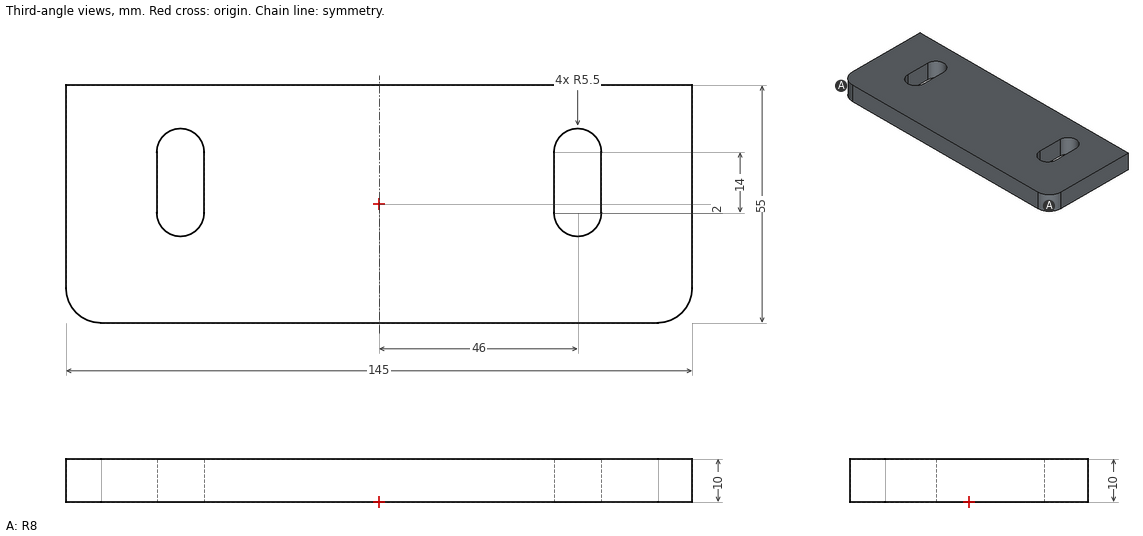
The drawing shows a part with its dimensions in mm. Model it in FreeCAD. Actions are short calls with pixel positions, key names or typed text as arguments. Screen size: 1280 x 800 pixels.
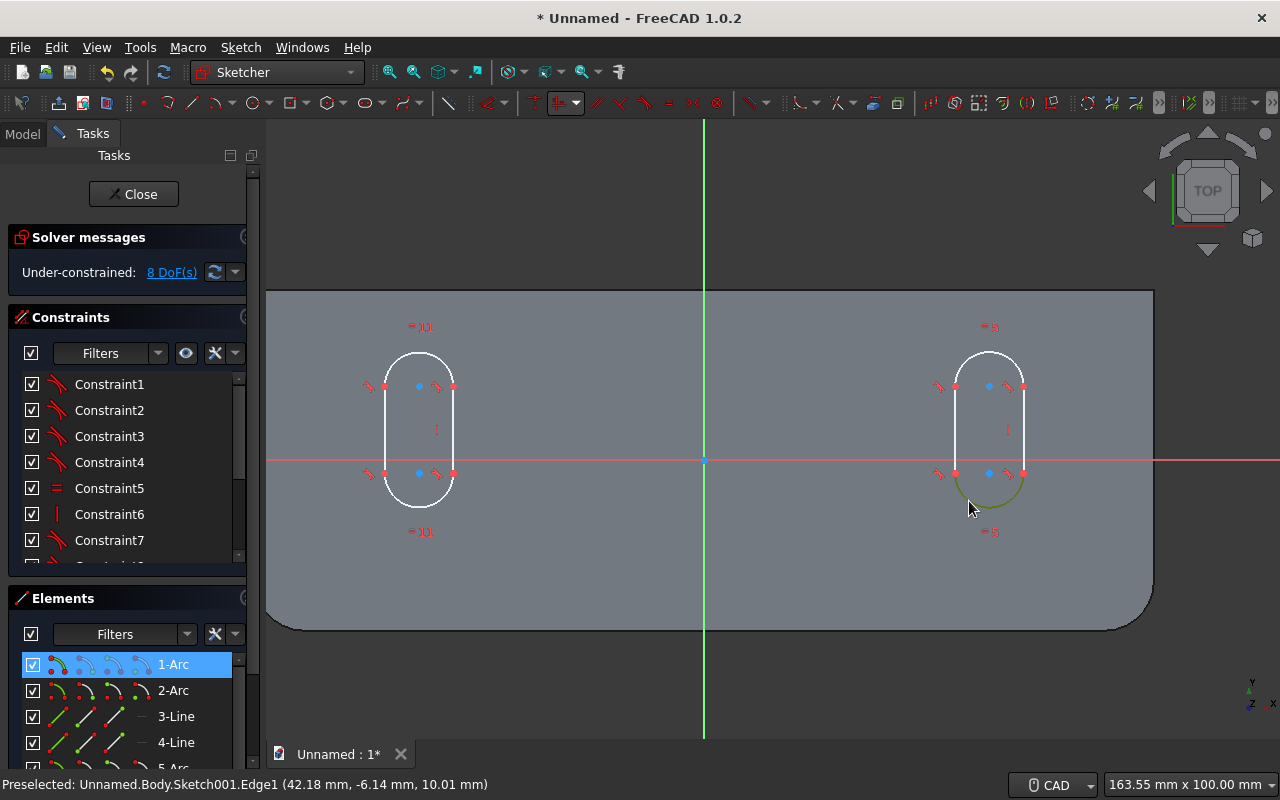
click(399, 501)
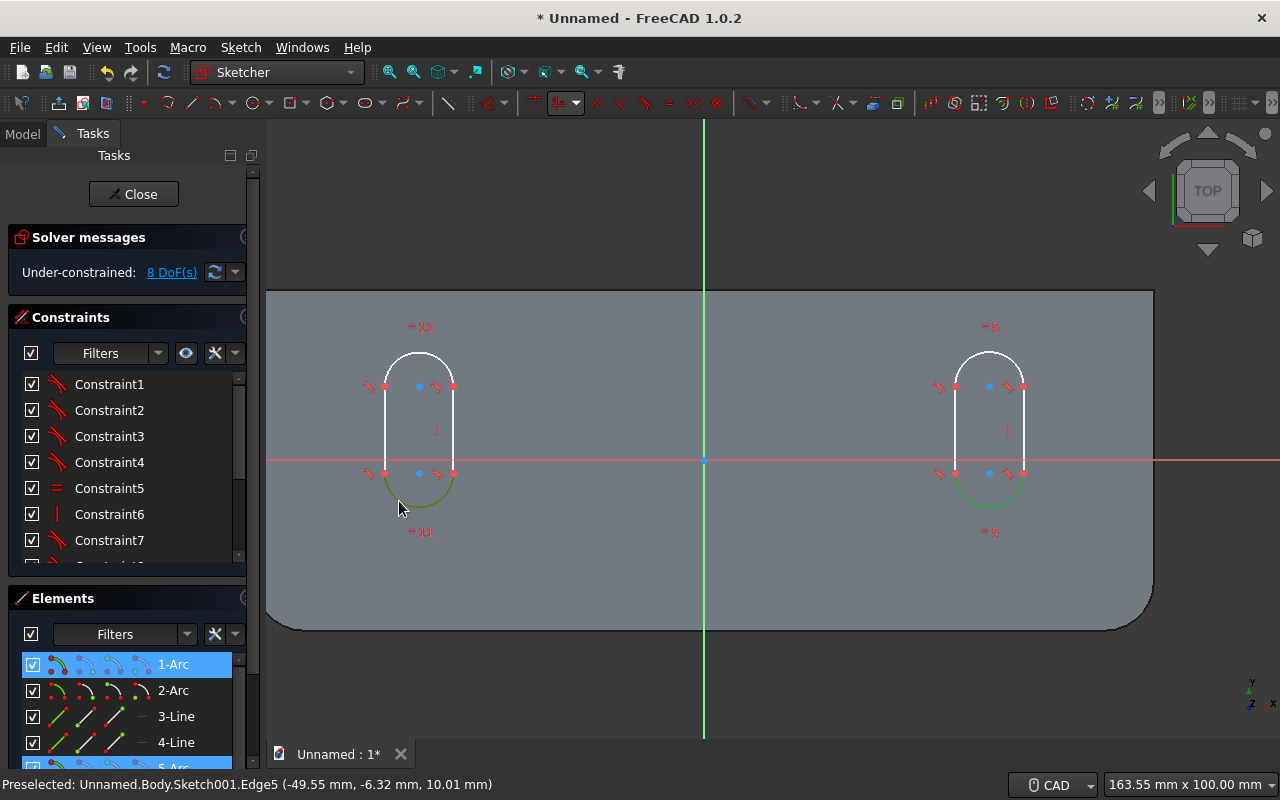
click(670, 104)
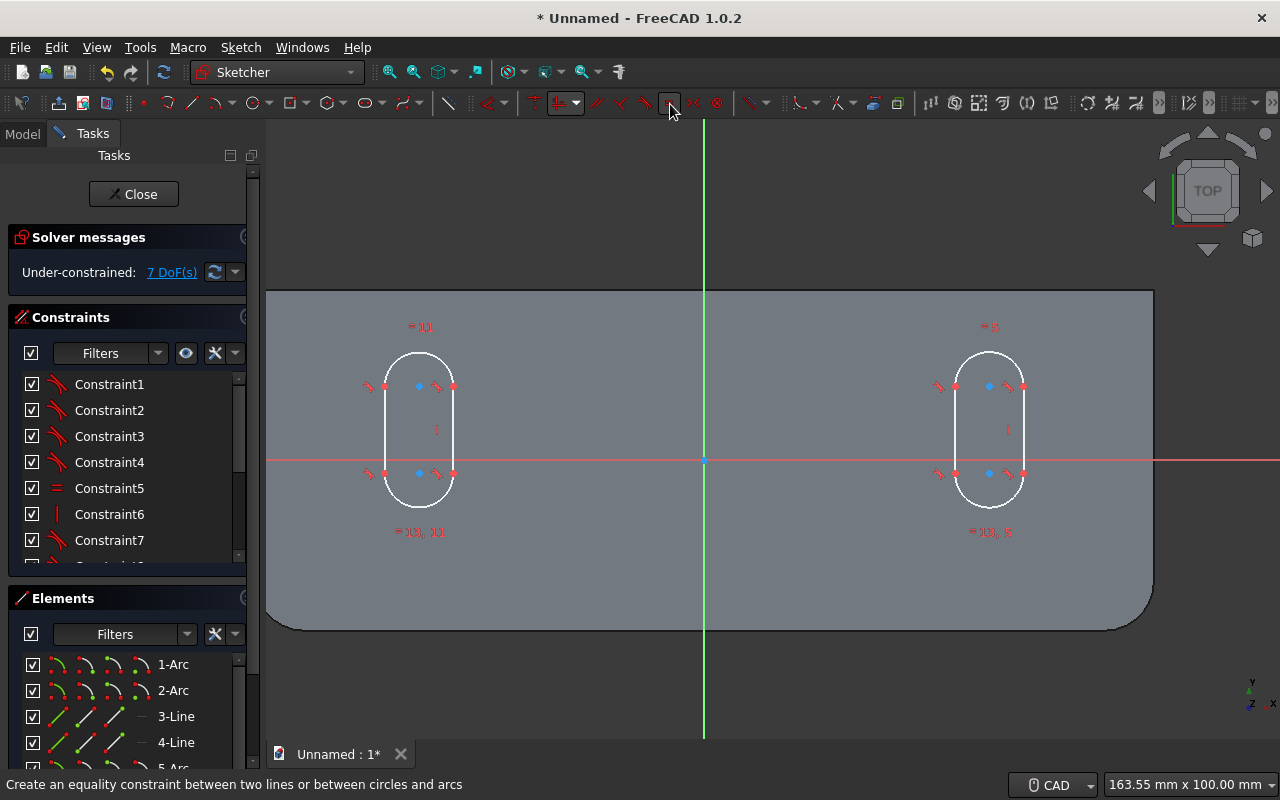
click(989, 473)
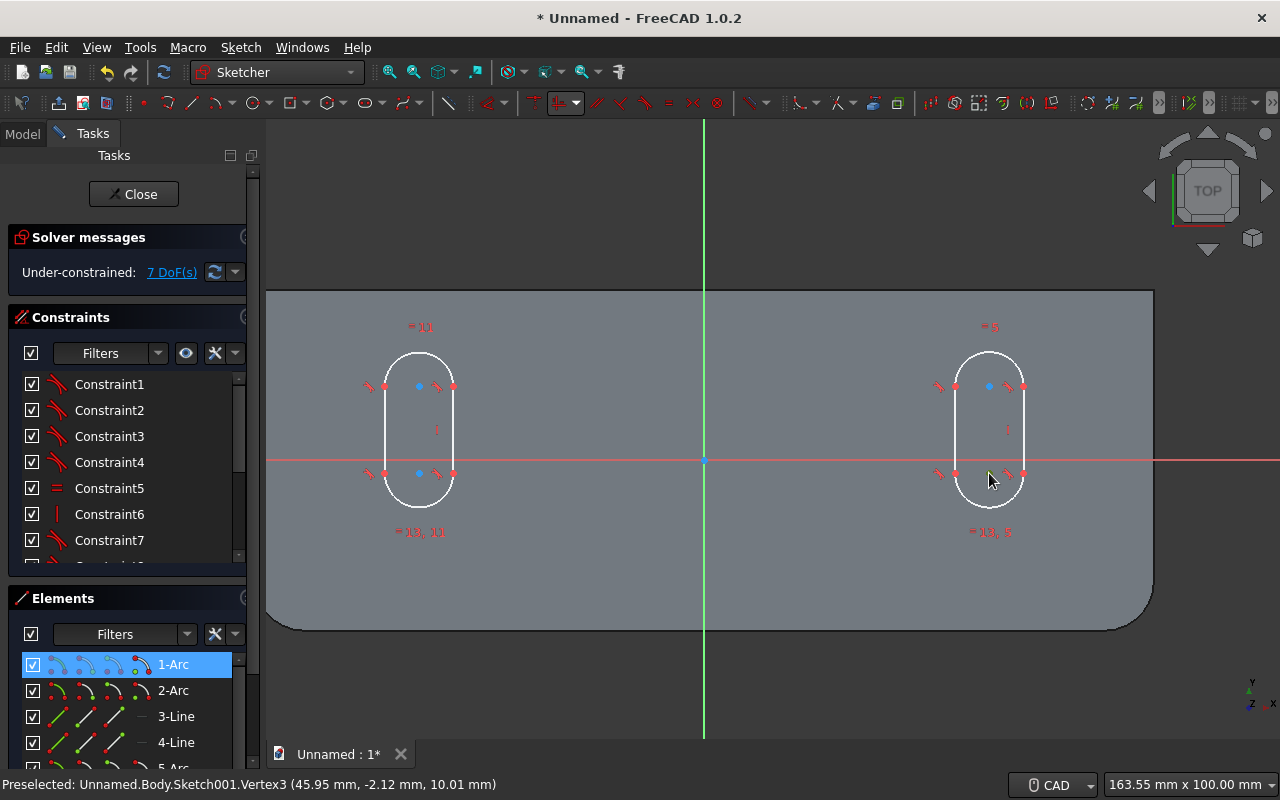
click(419, 473)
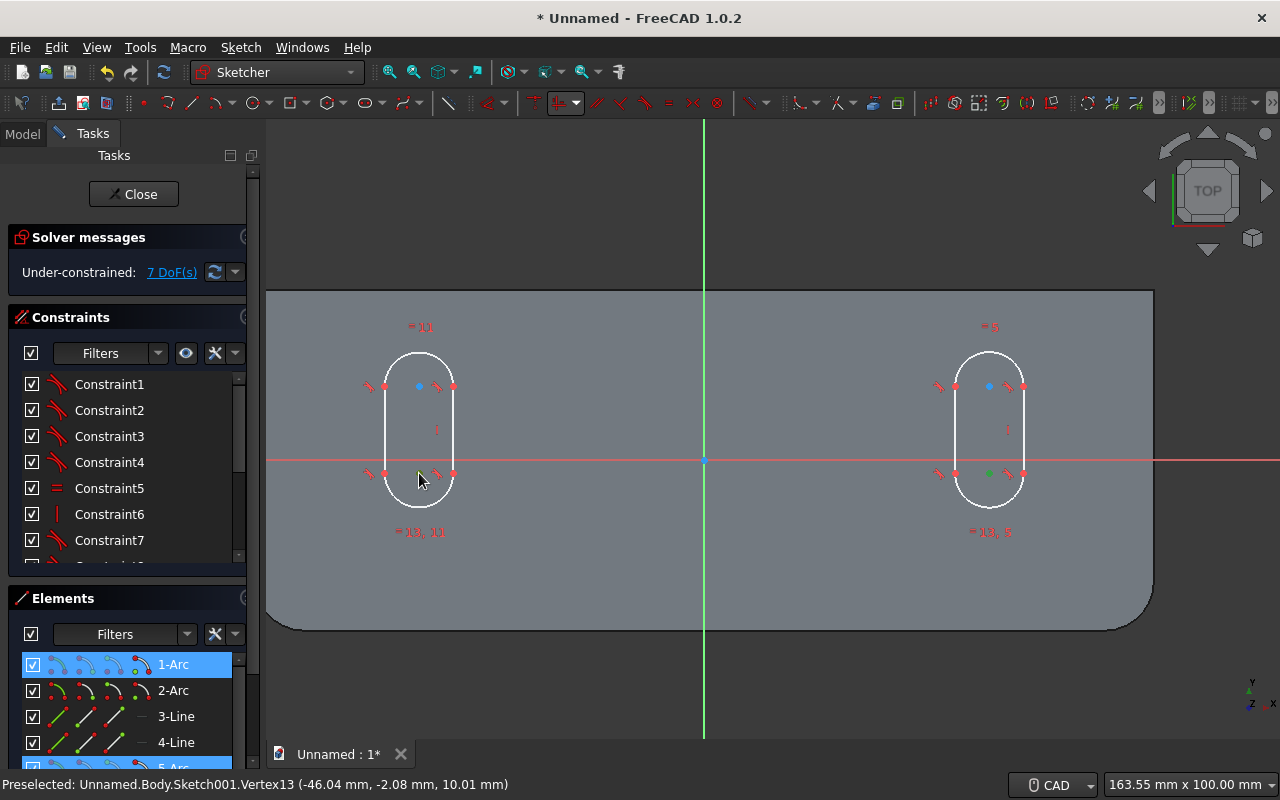
click(704, 671)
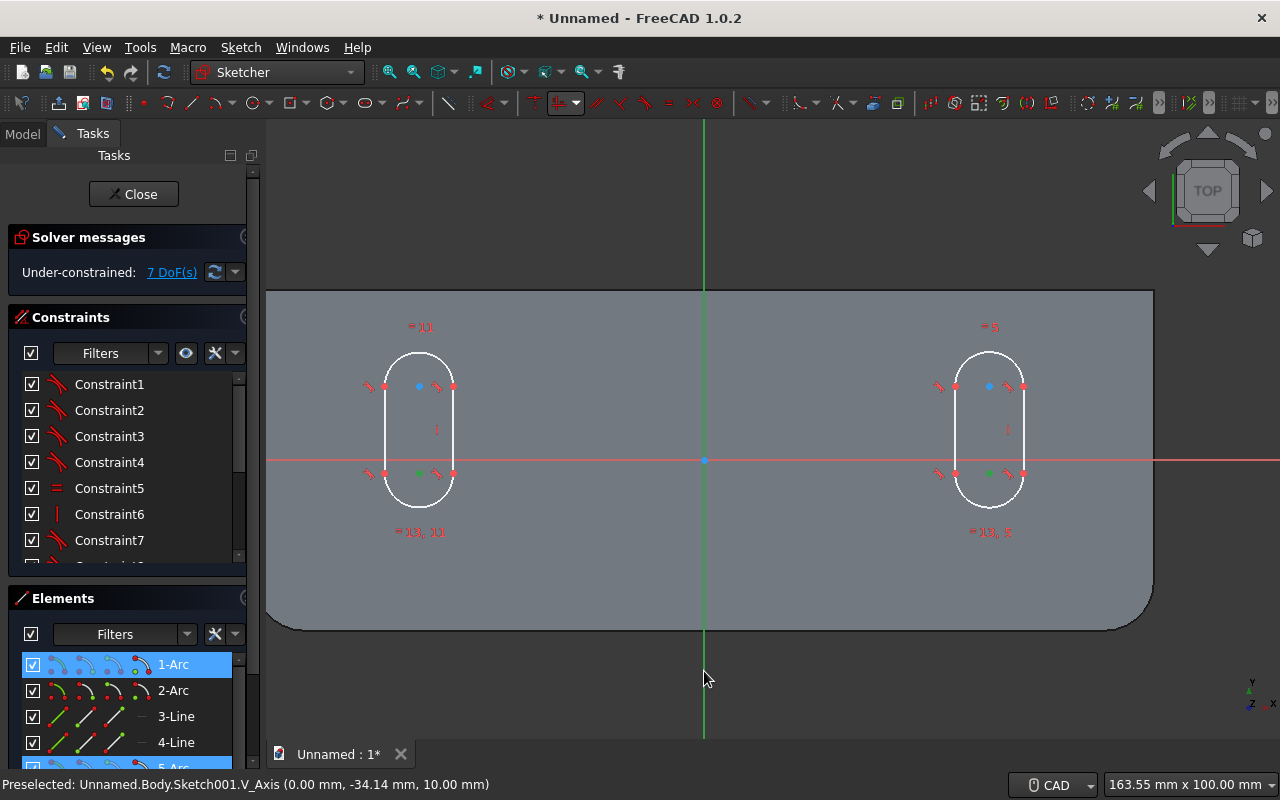
click(694, 104)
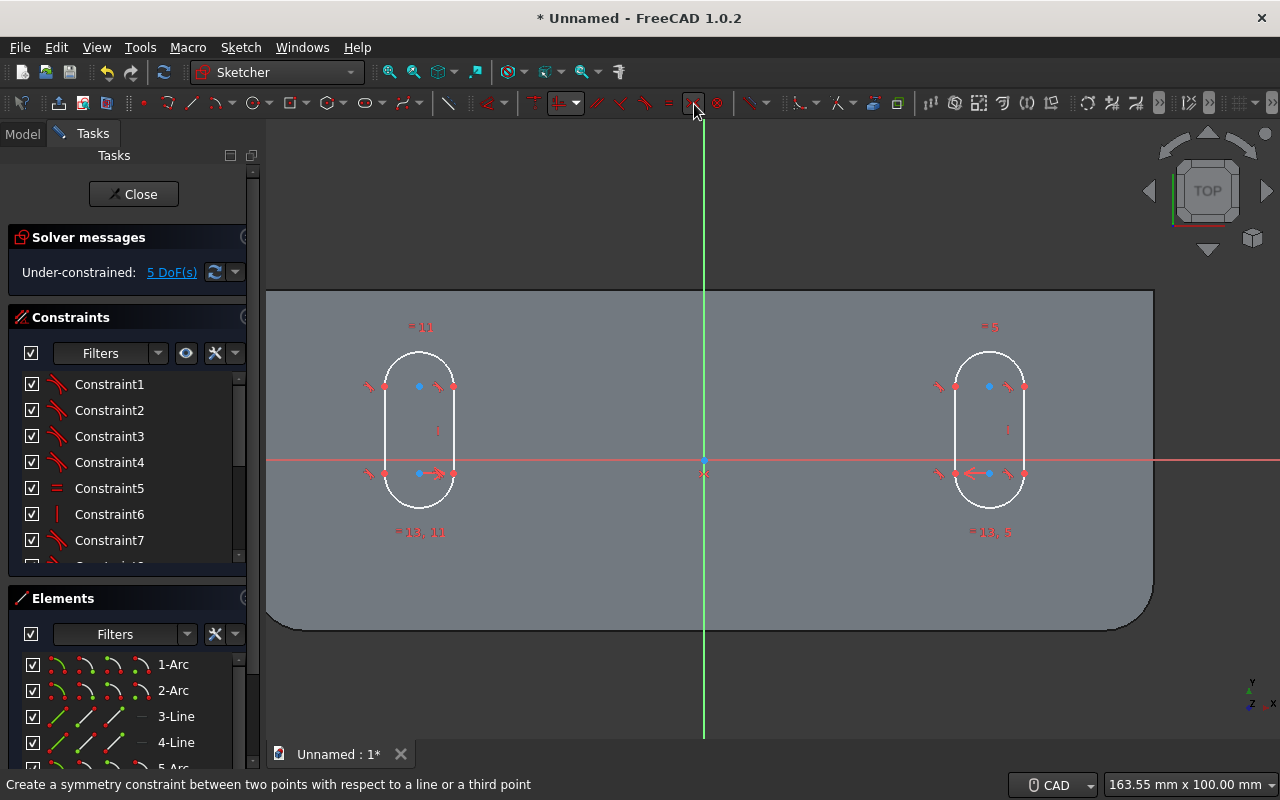
click(488, 104)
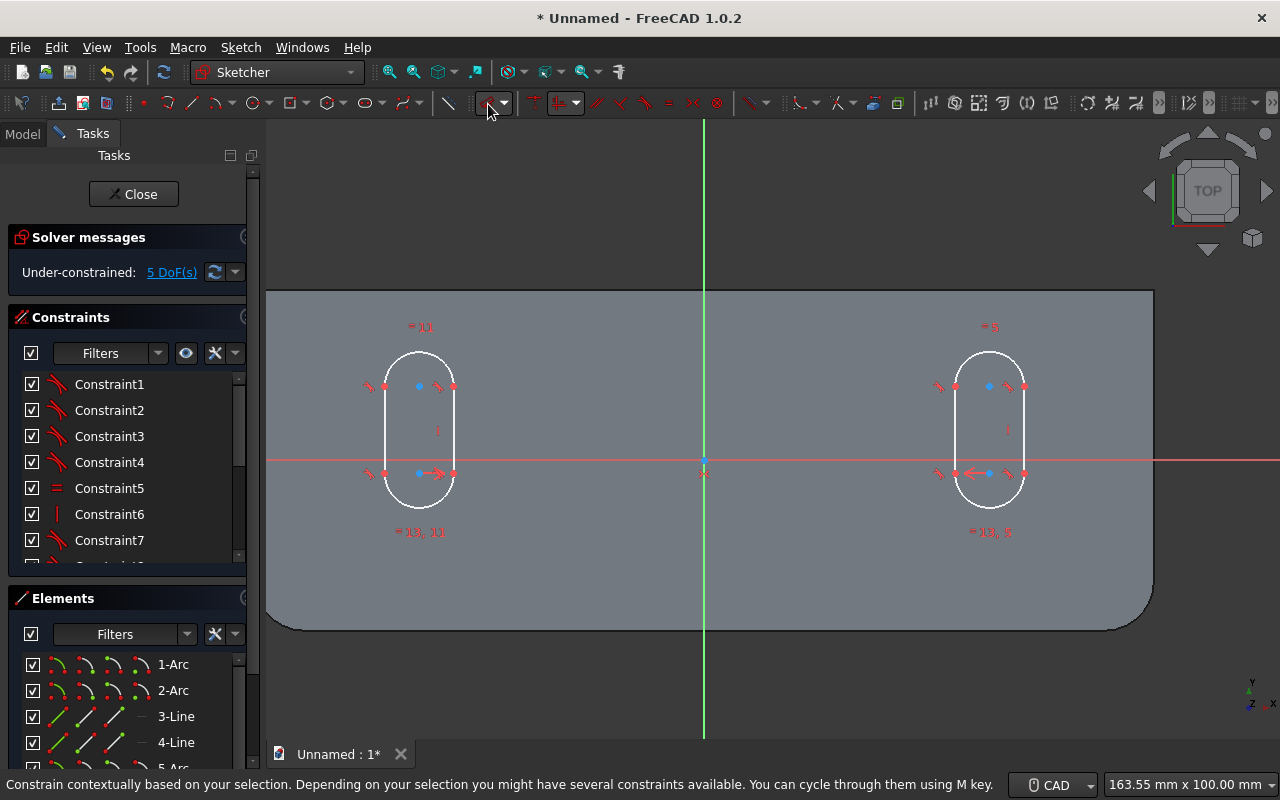
click(969, 501)
click(950, 527)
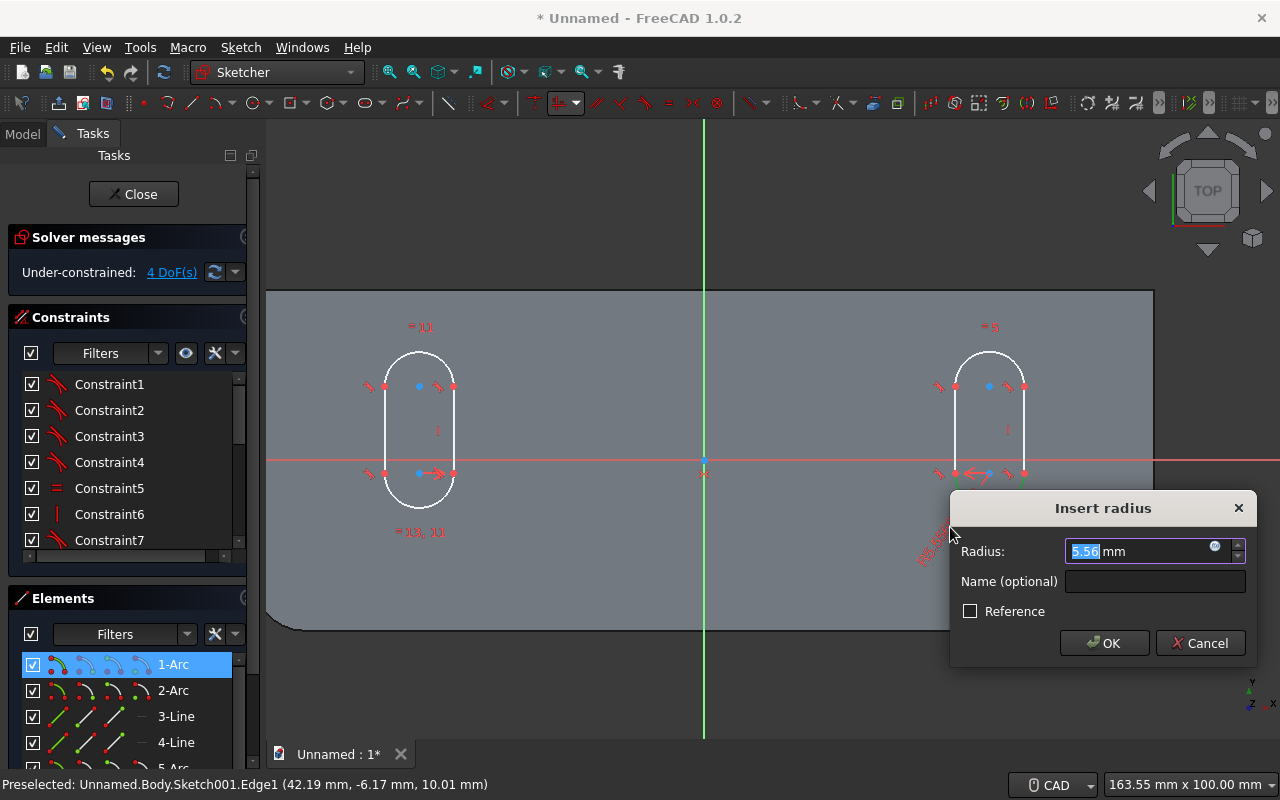
text(5.5)
key(Return)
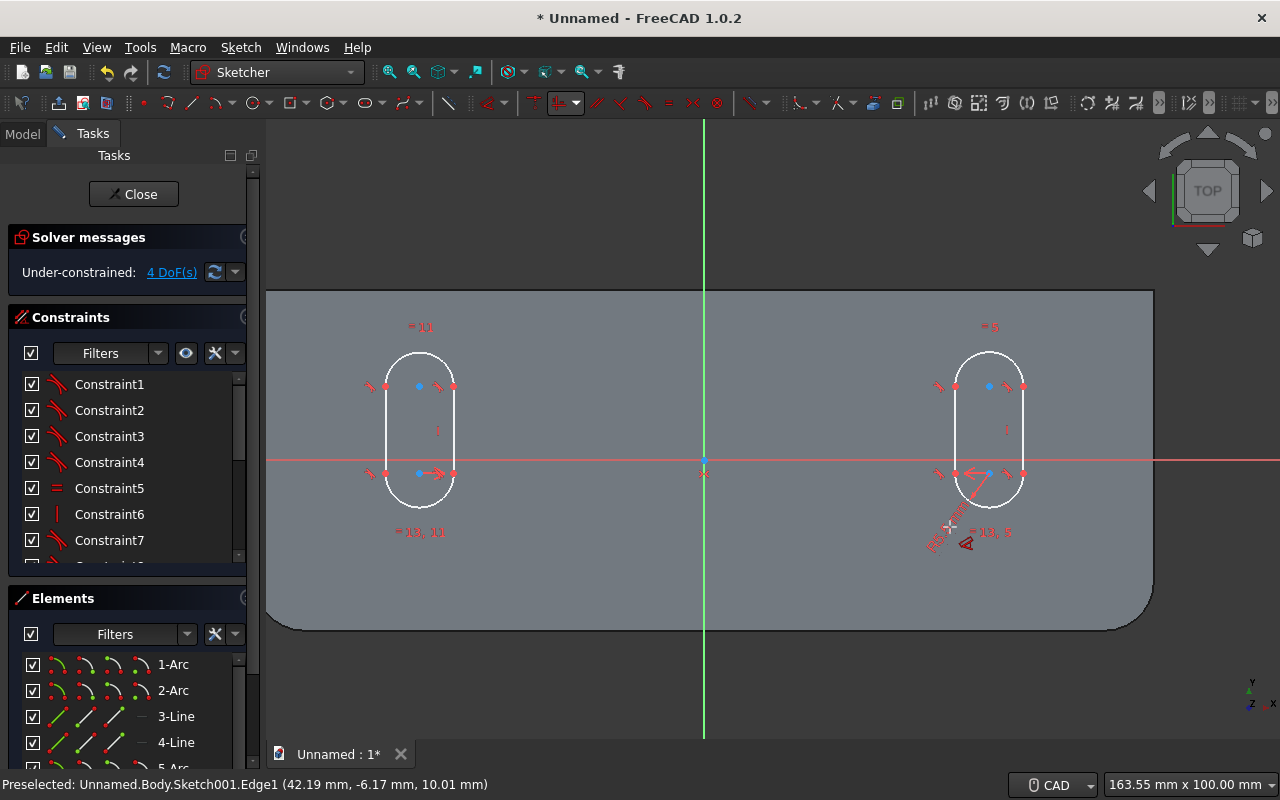
click(955, 447)
click(989, 430)